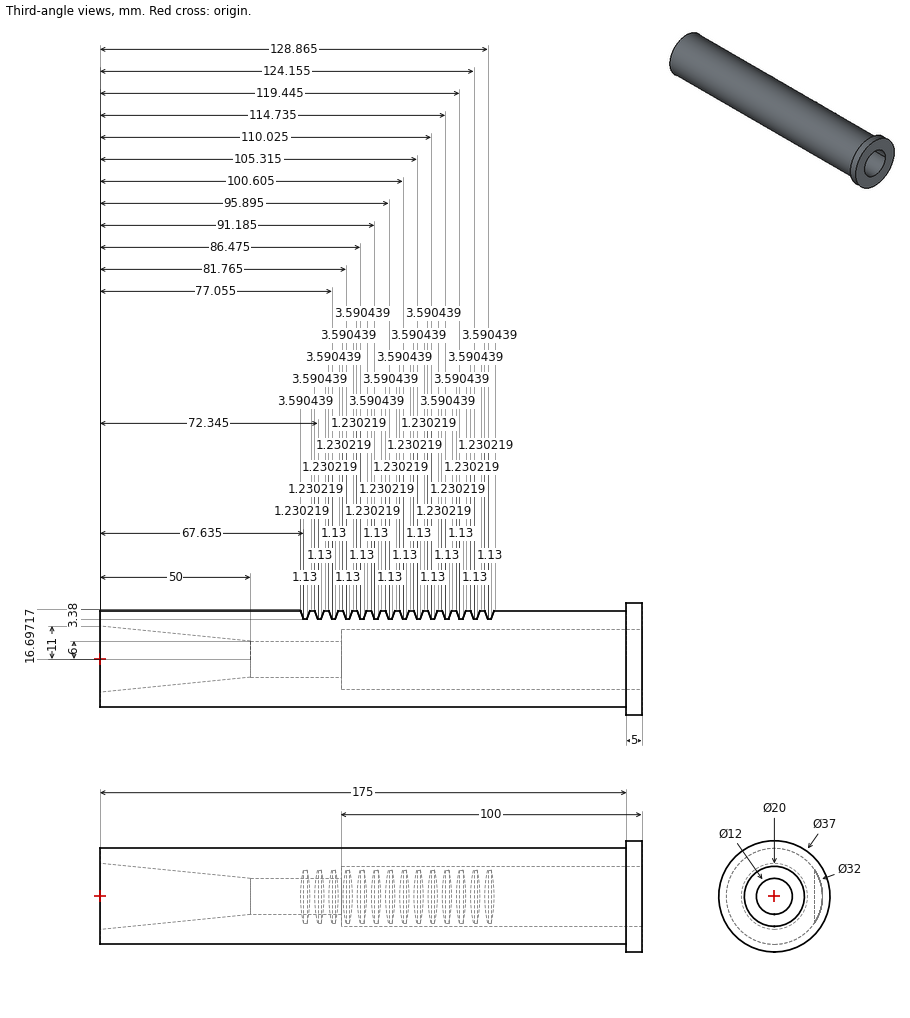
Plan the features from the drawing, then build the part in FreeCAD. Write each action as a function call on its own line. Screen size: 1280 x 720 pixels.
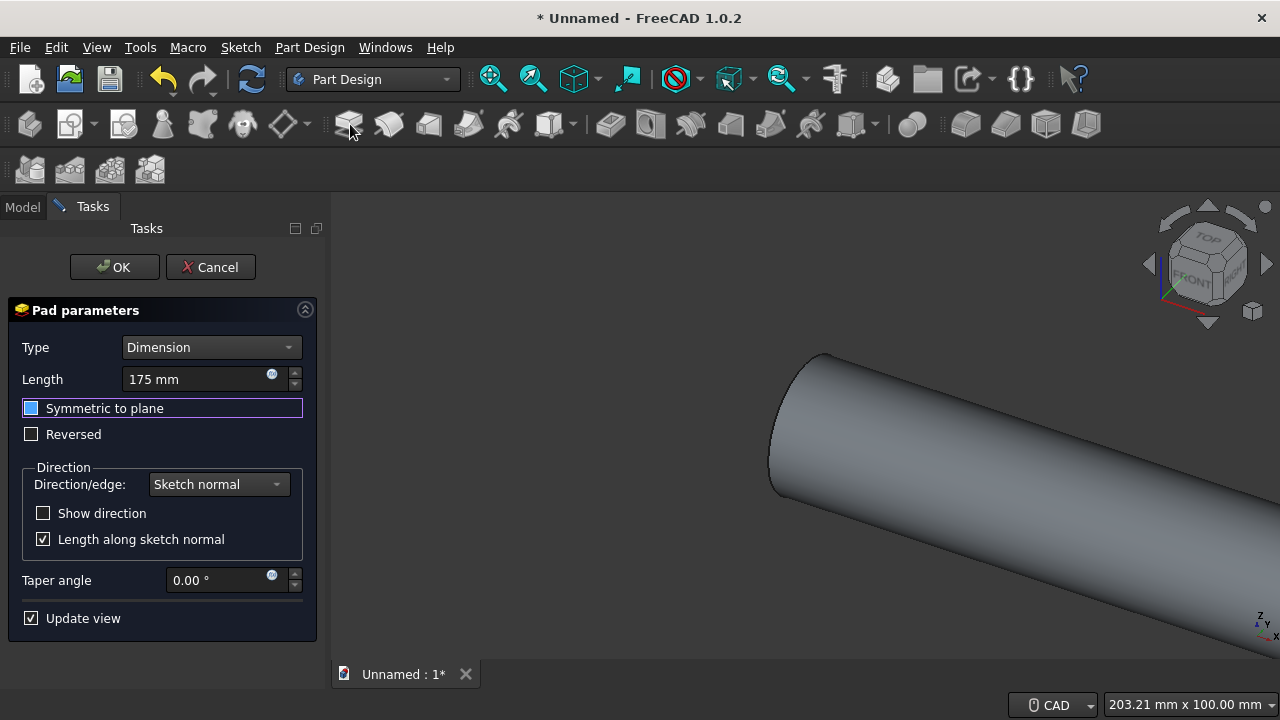
click(115, 267)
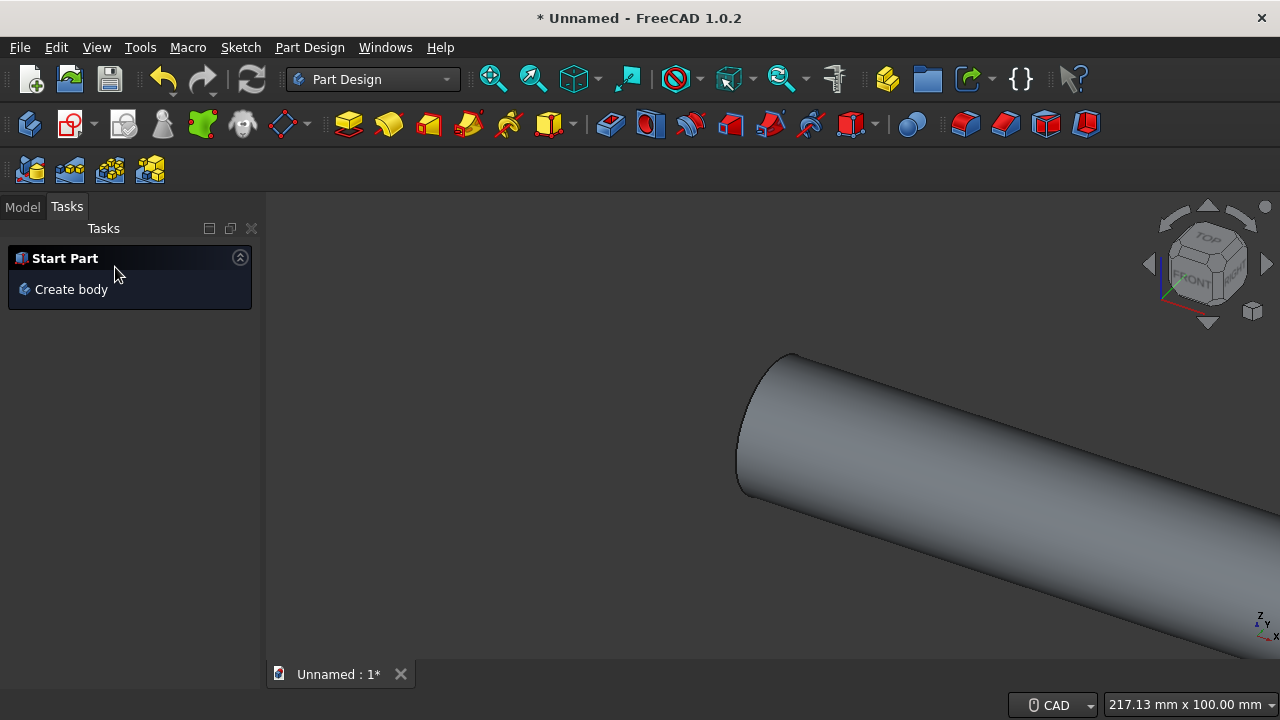
click(494, 80)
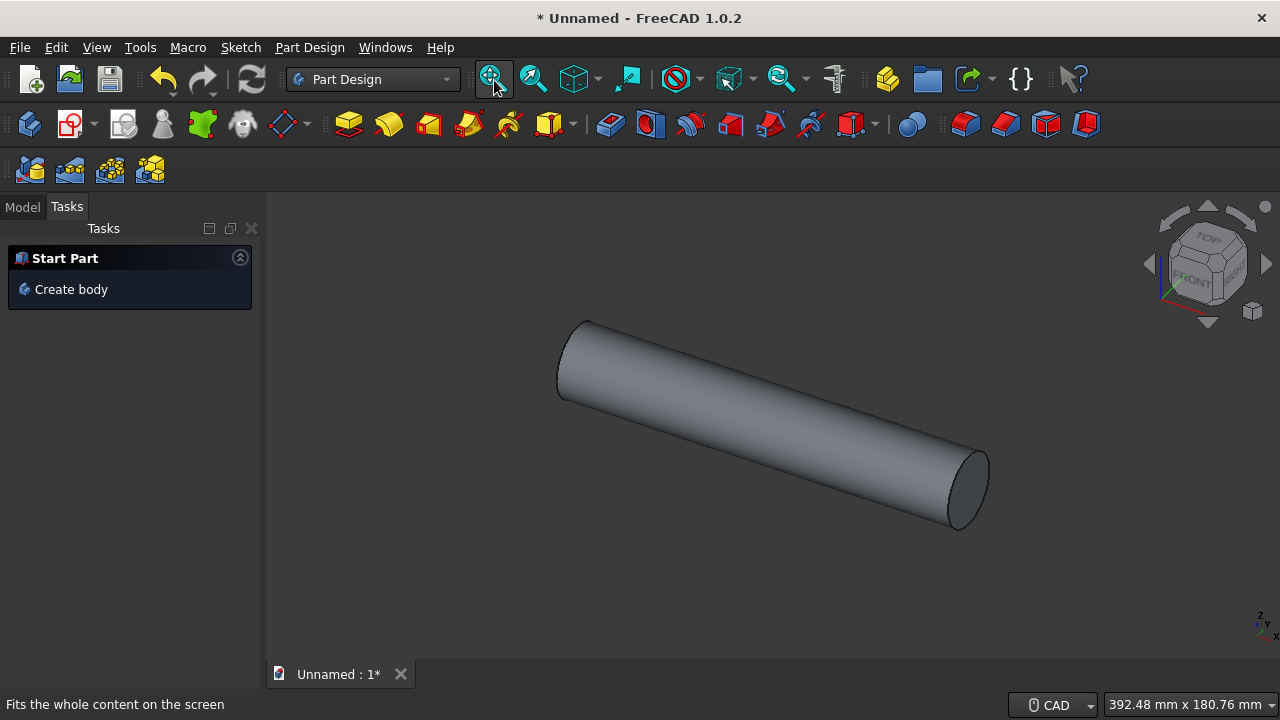
click(969, 489)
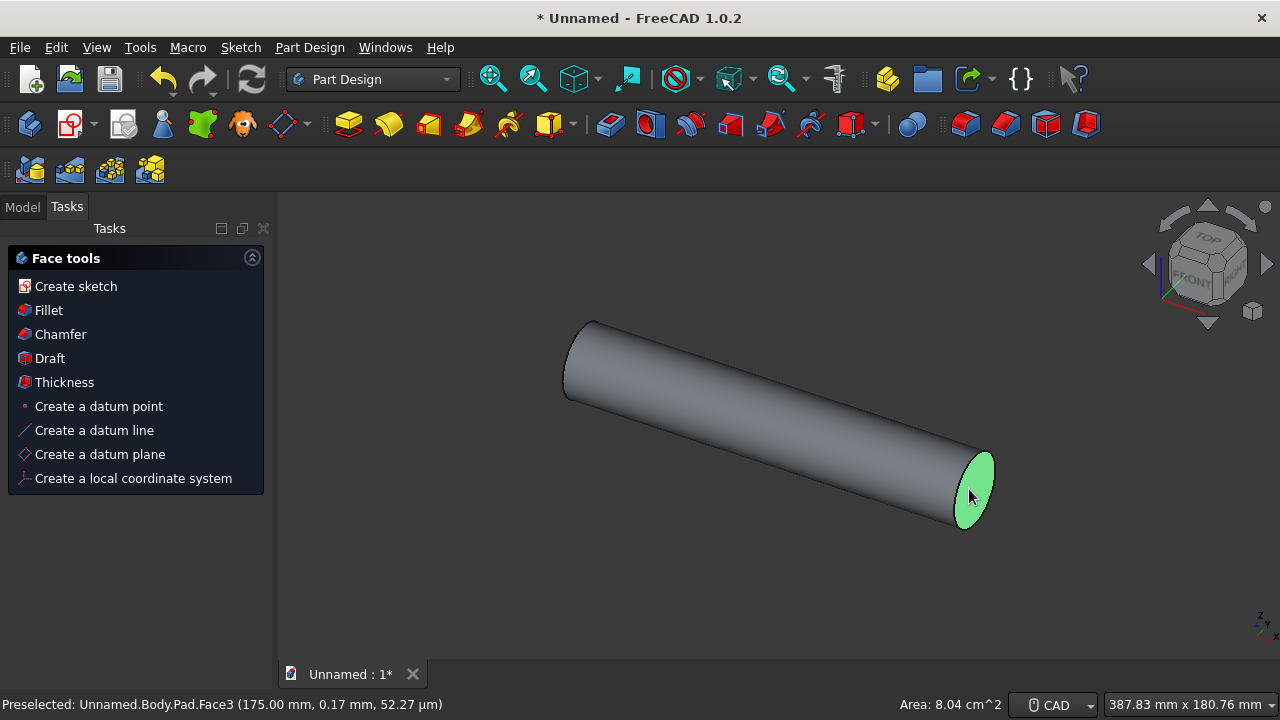
click(70, 124)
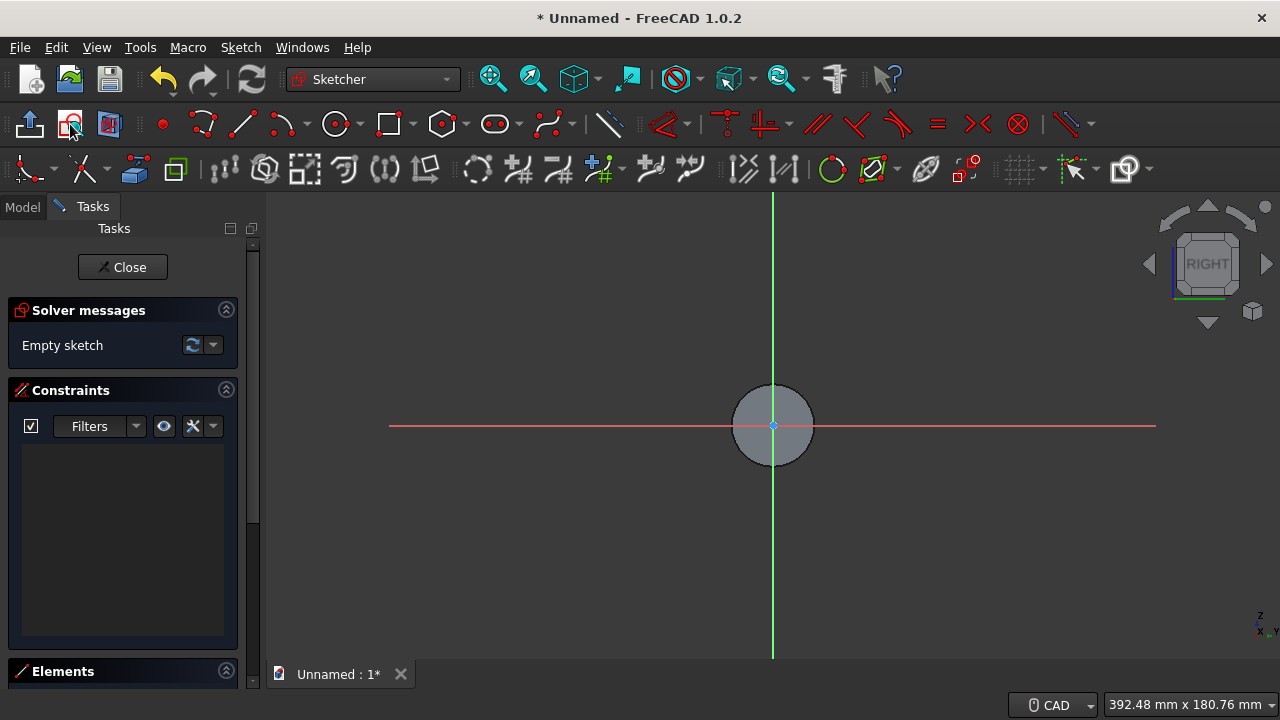
scroll(803, 425, up, 6)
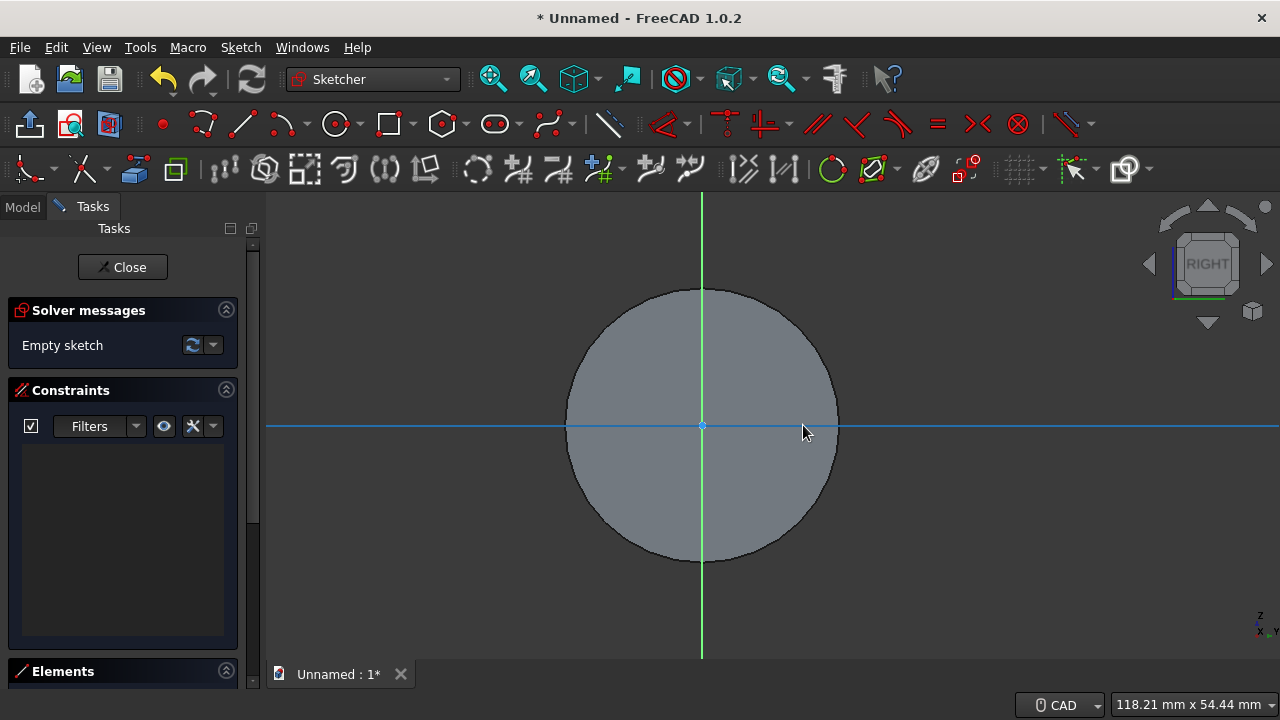
key(g)
key(c)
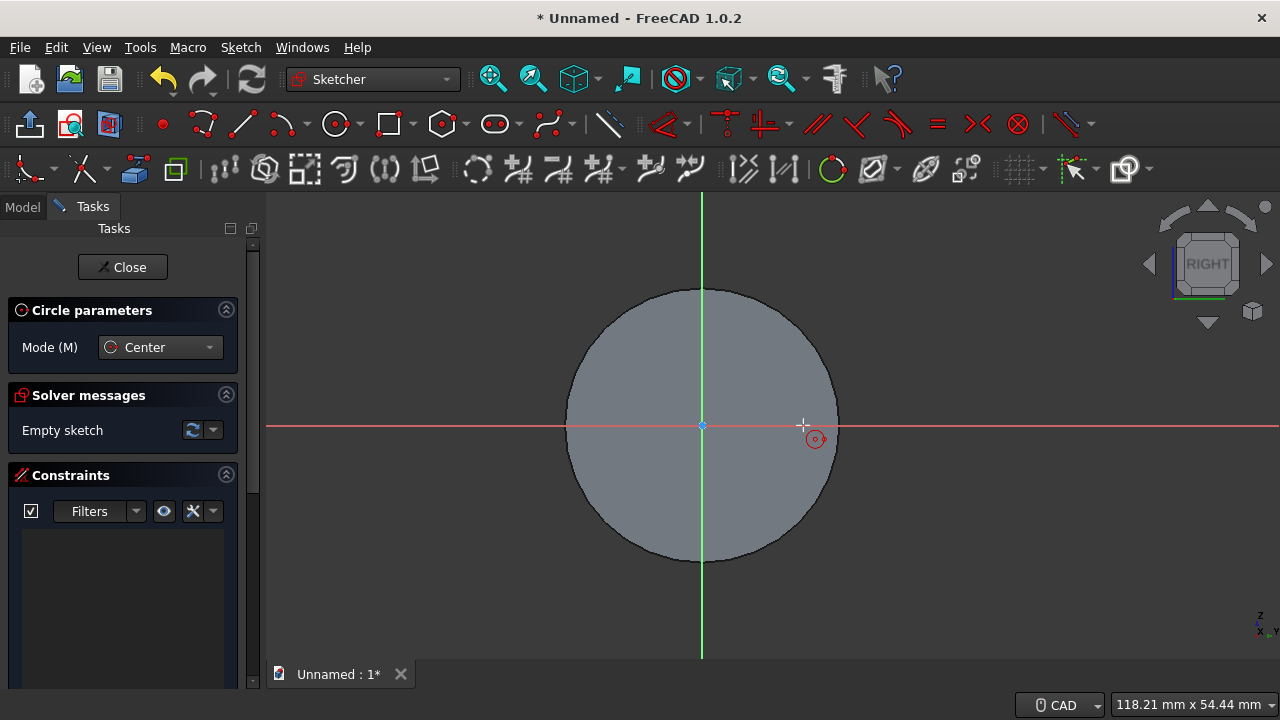
click(702, 425)
move(814, 313)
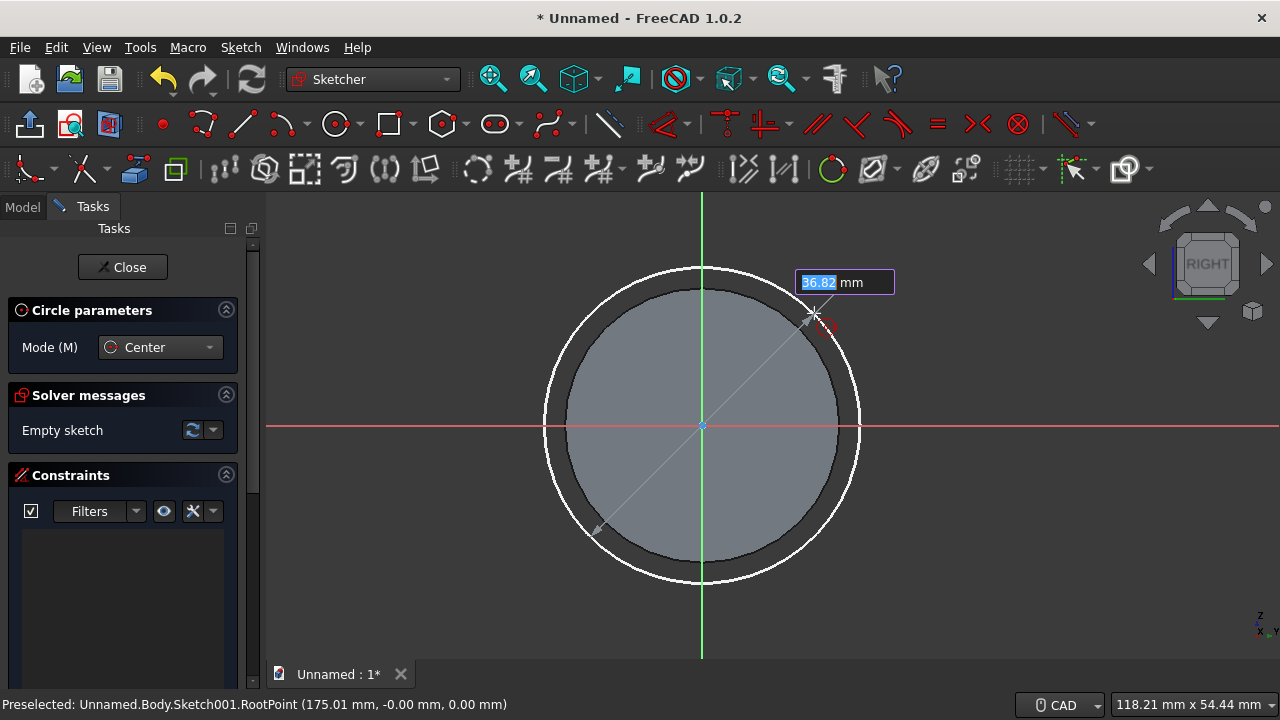
text(37)
key(Return)
key(Escape)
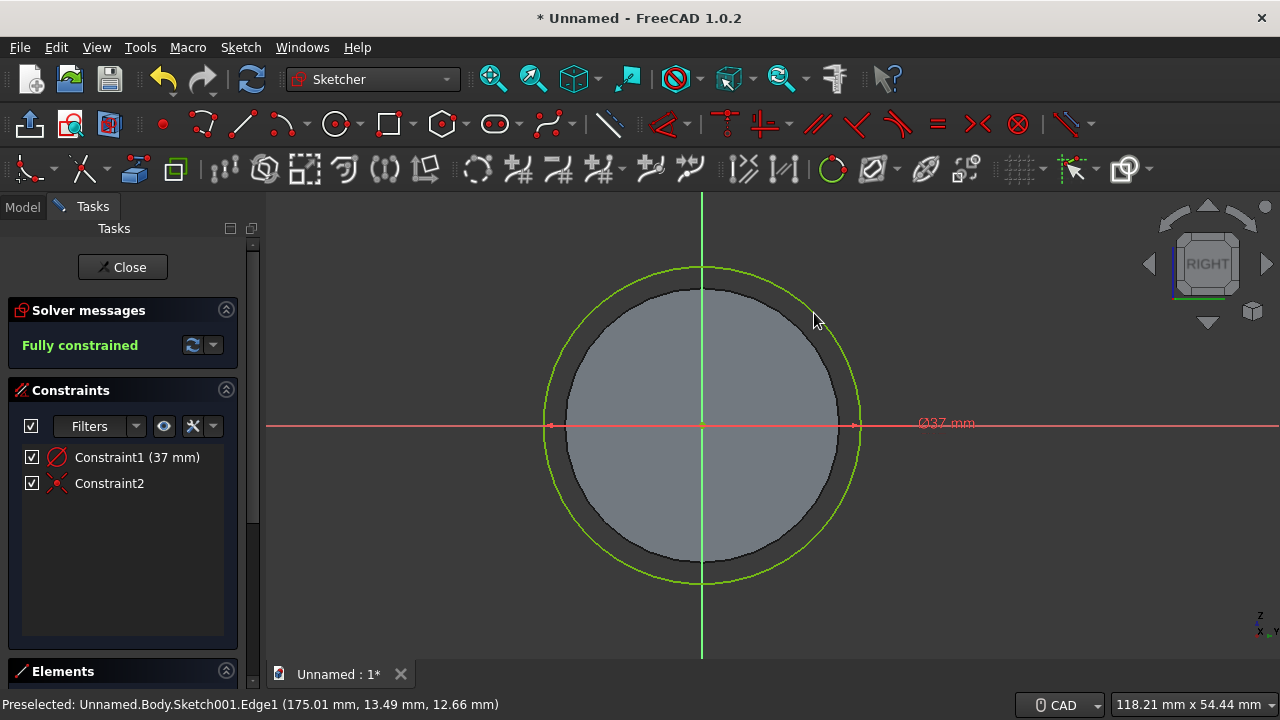
click(123, 267)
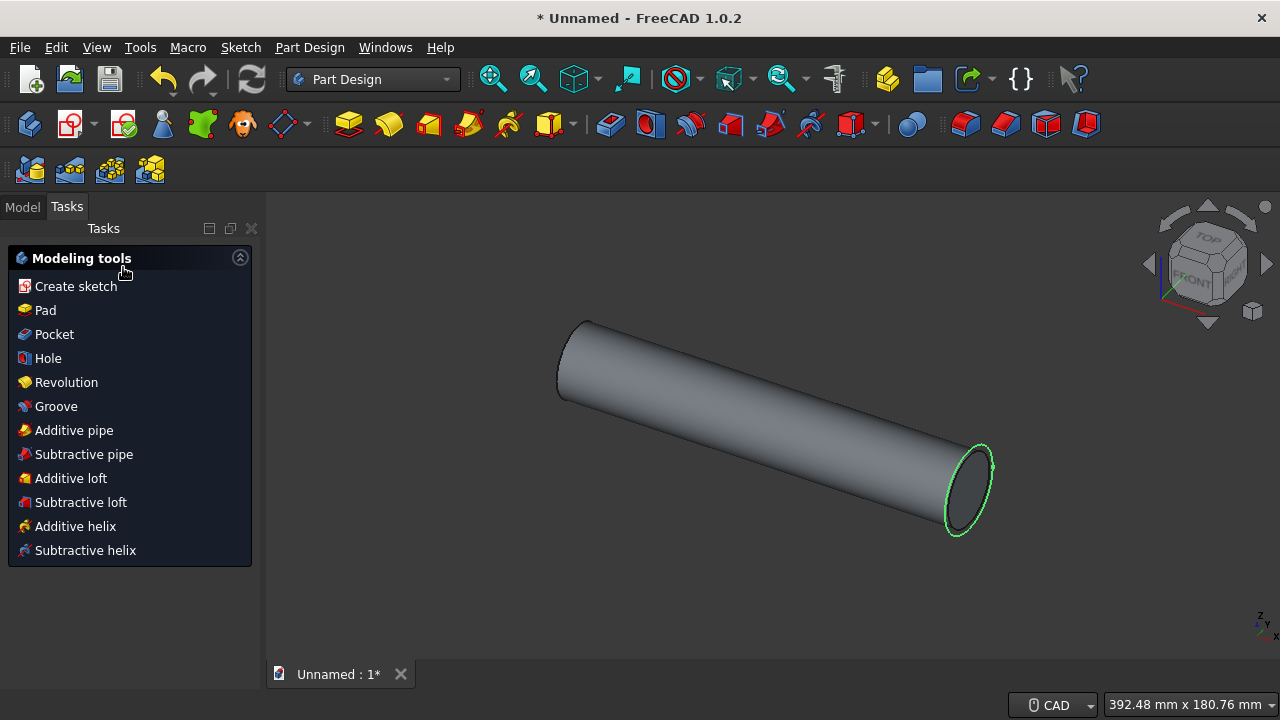
click(350, 124)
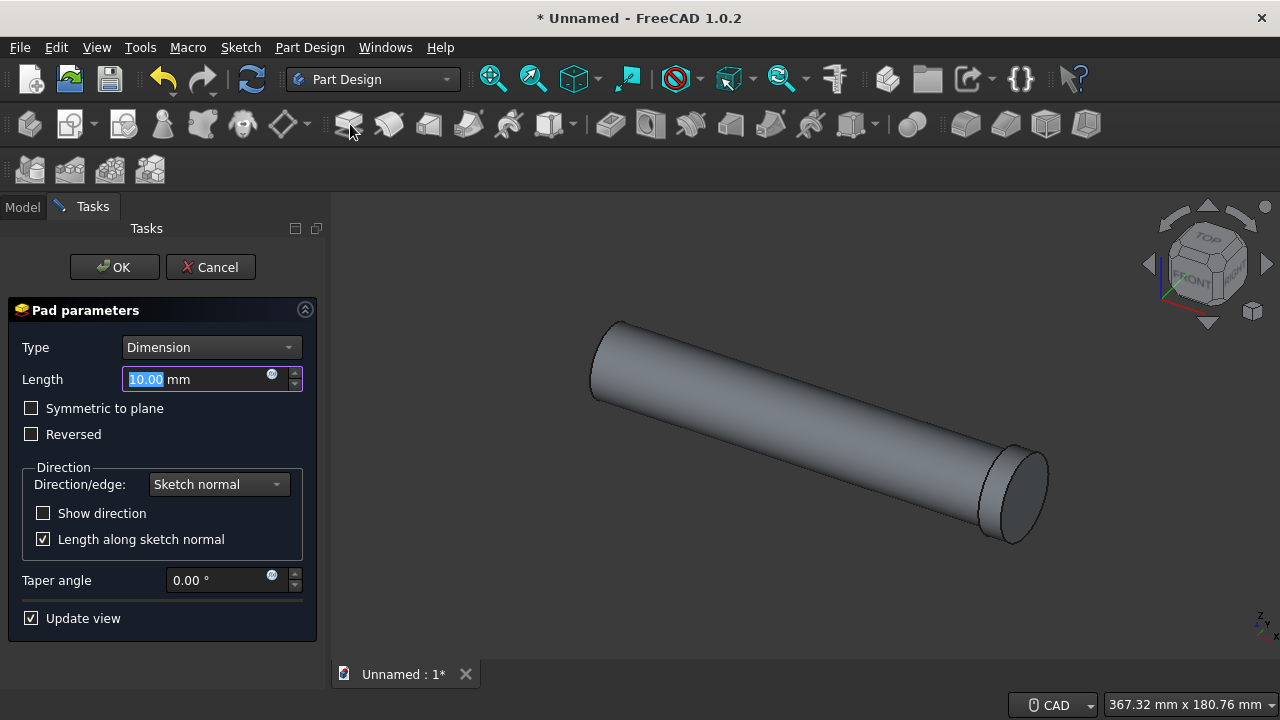
text(5)
key(Tab)